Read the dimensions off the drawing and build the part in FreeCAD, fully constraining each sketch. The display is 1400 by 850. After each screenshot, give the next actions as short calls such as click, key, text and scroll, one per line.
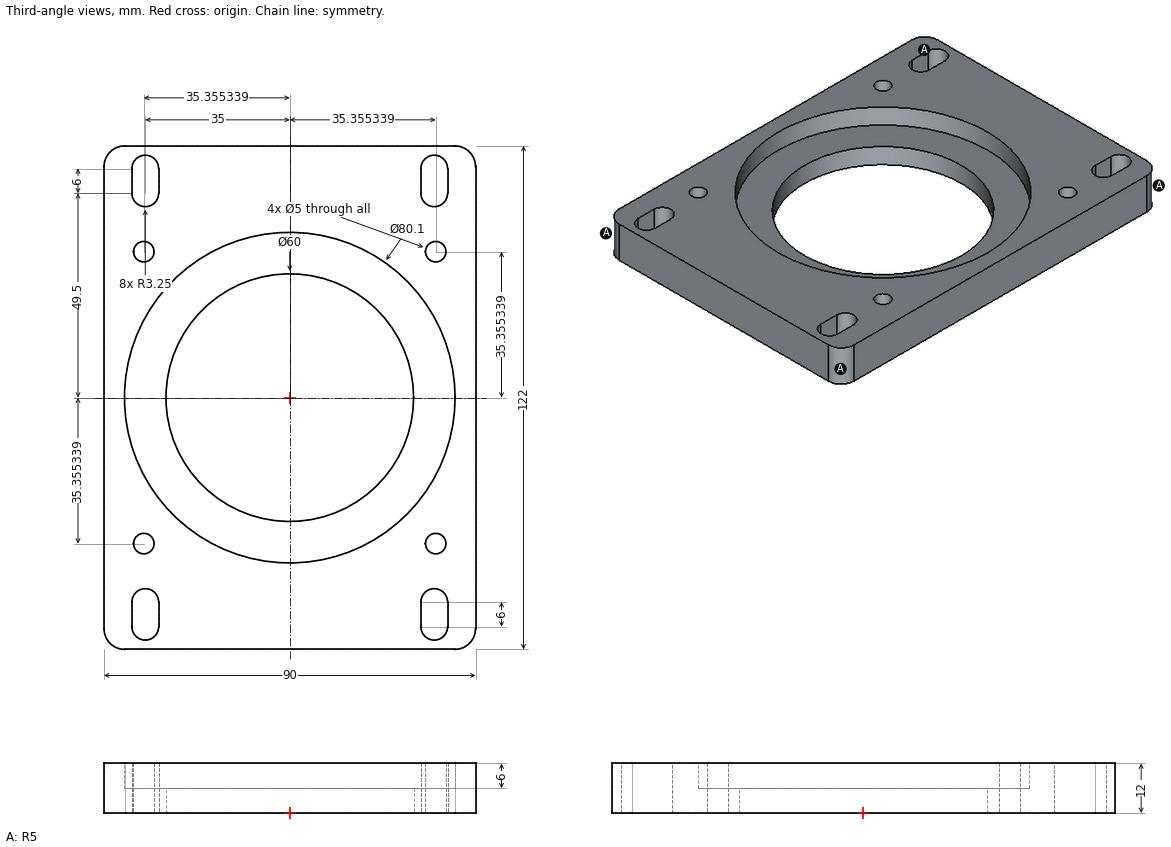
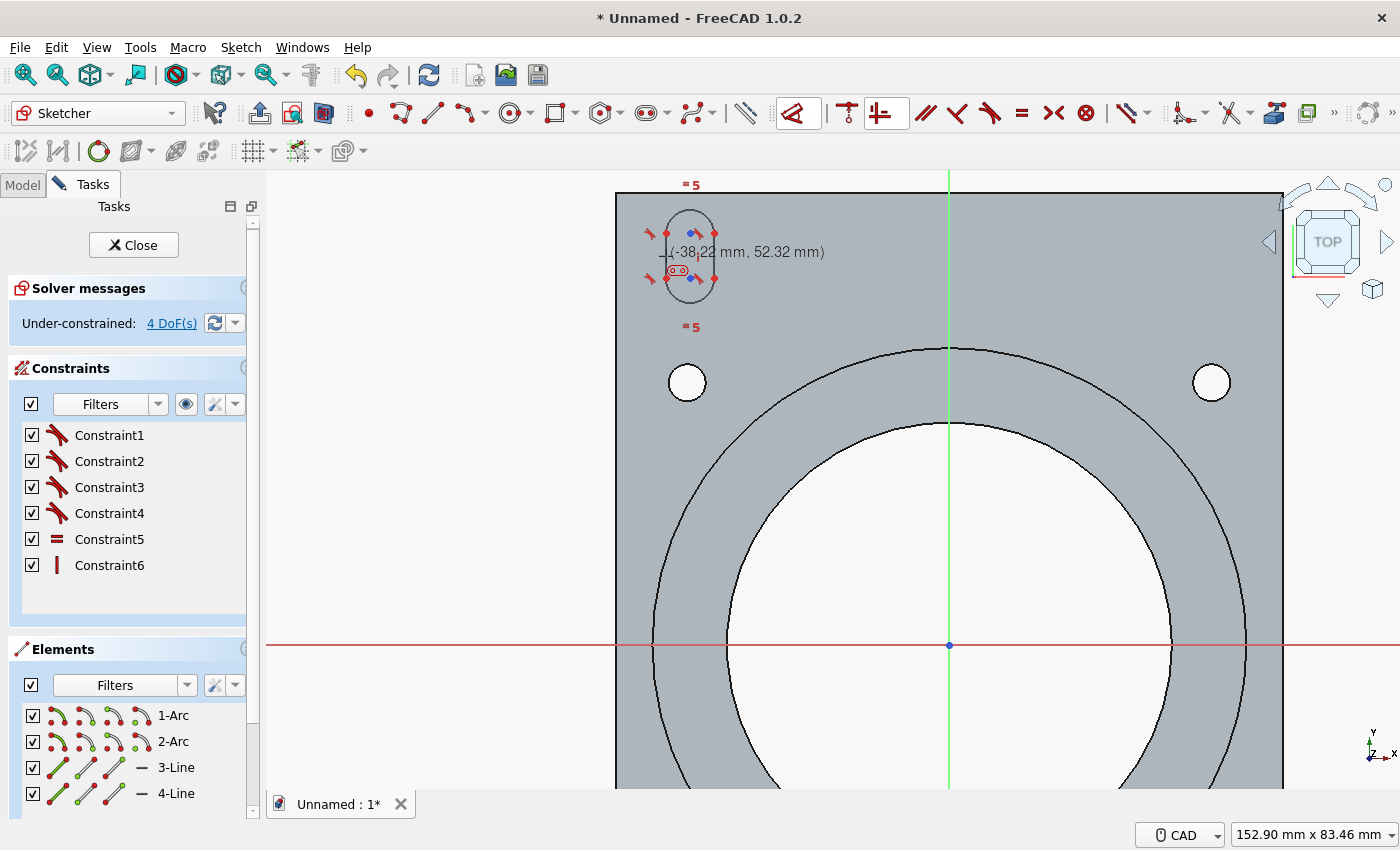
click(1209, 278)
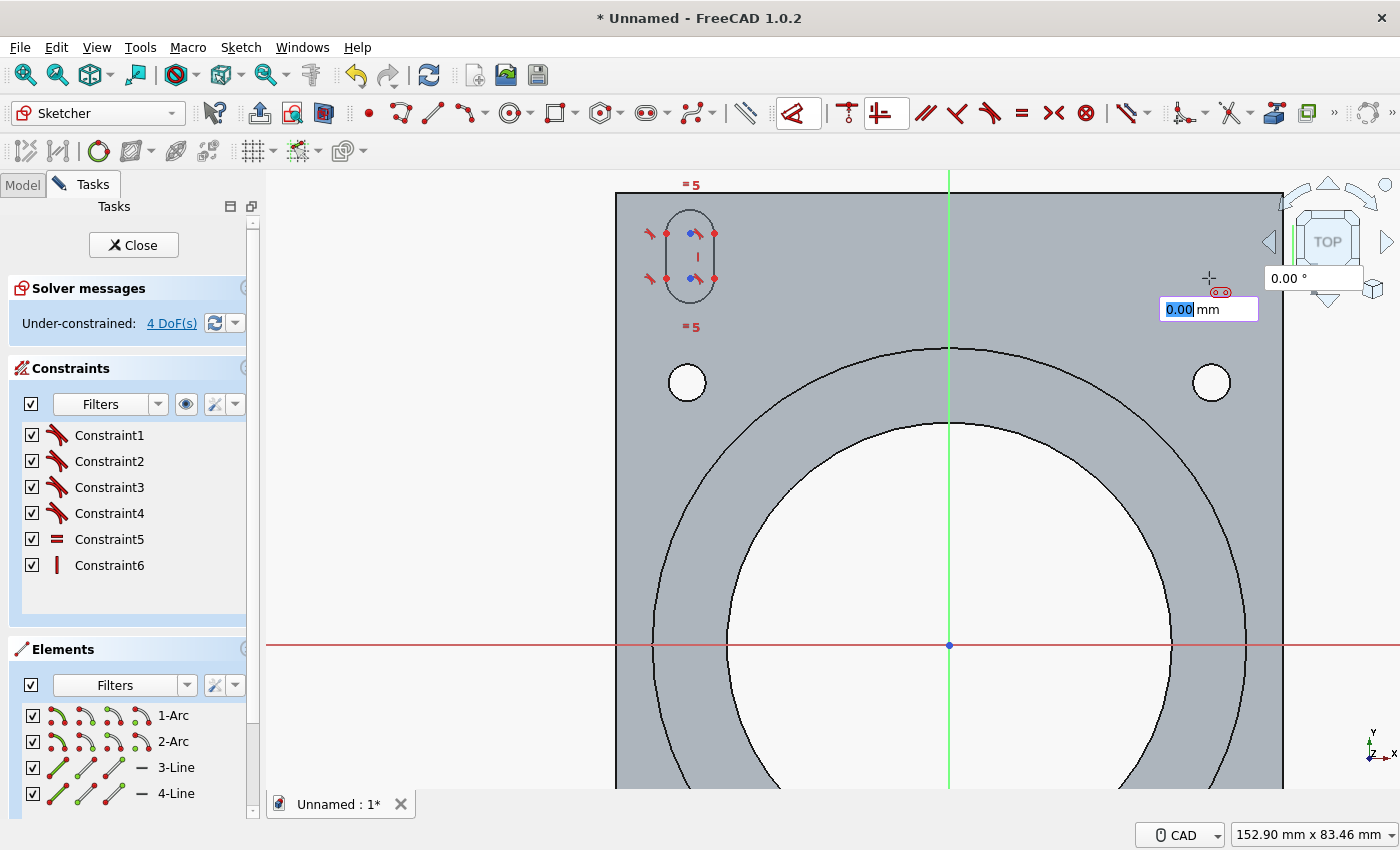
click(1209, 233)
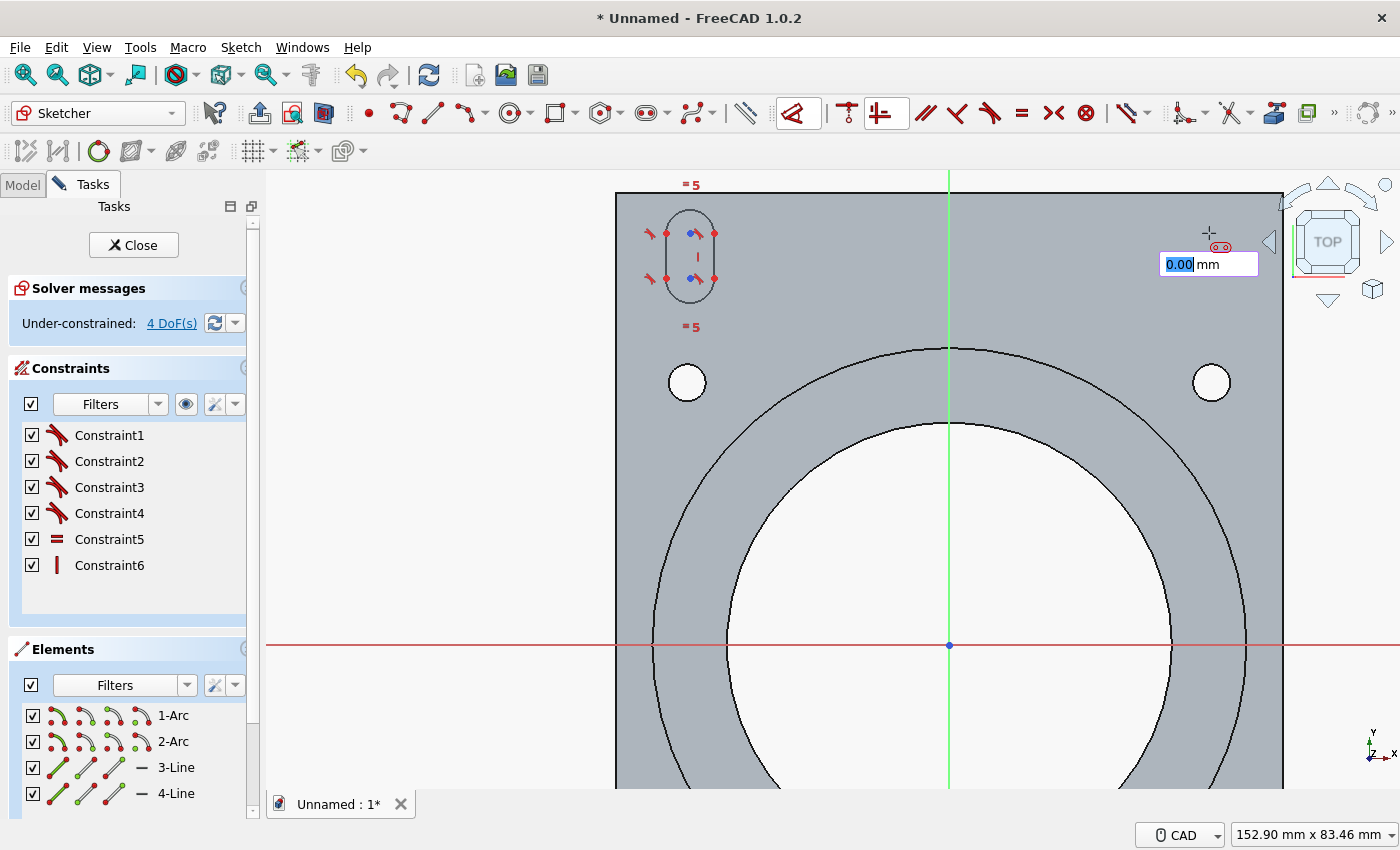
click(1233, 256)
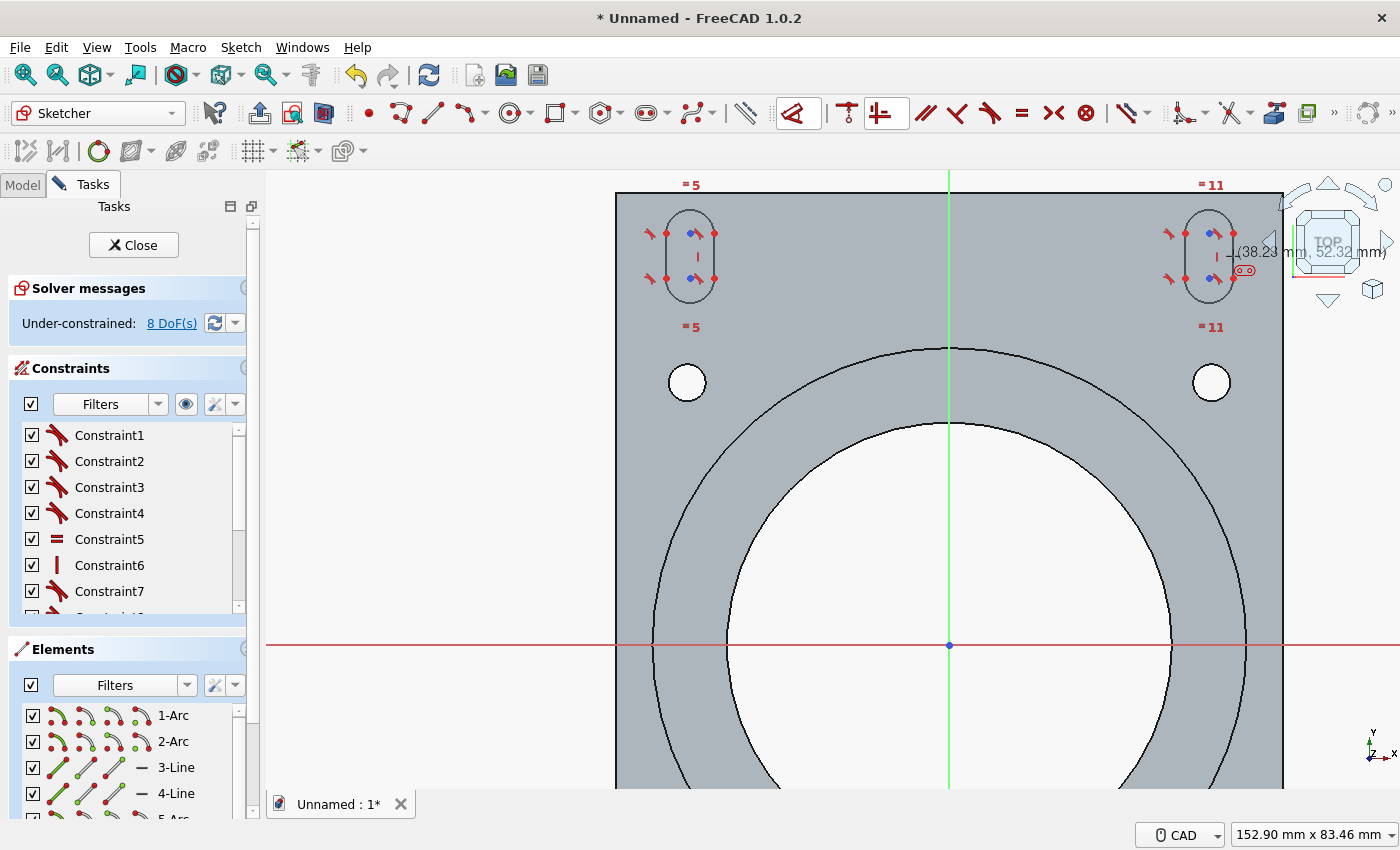
scroll(614, 344, down, 4)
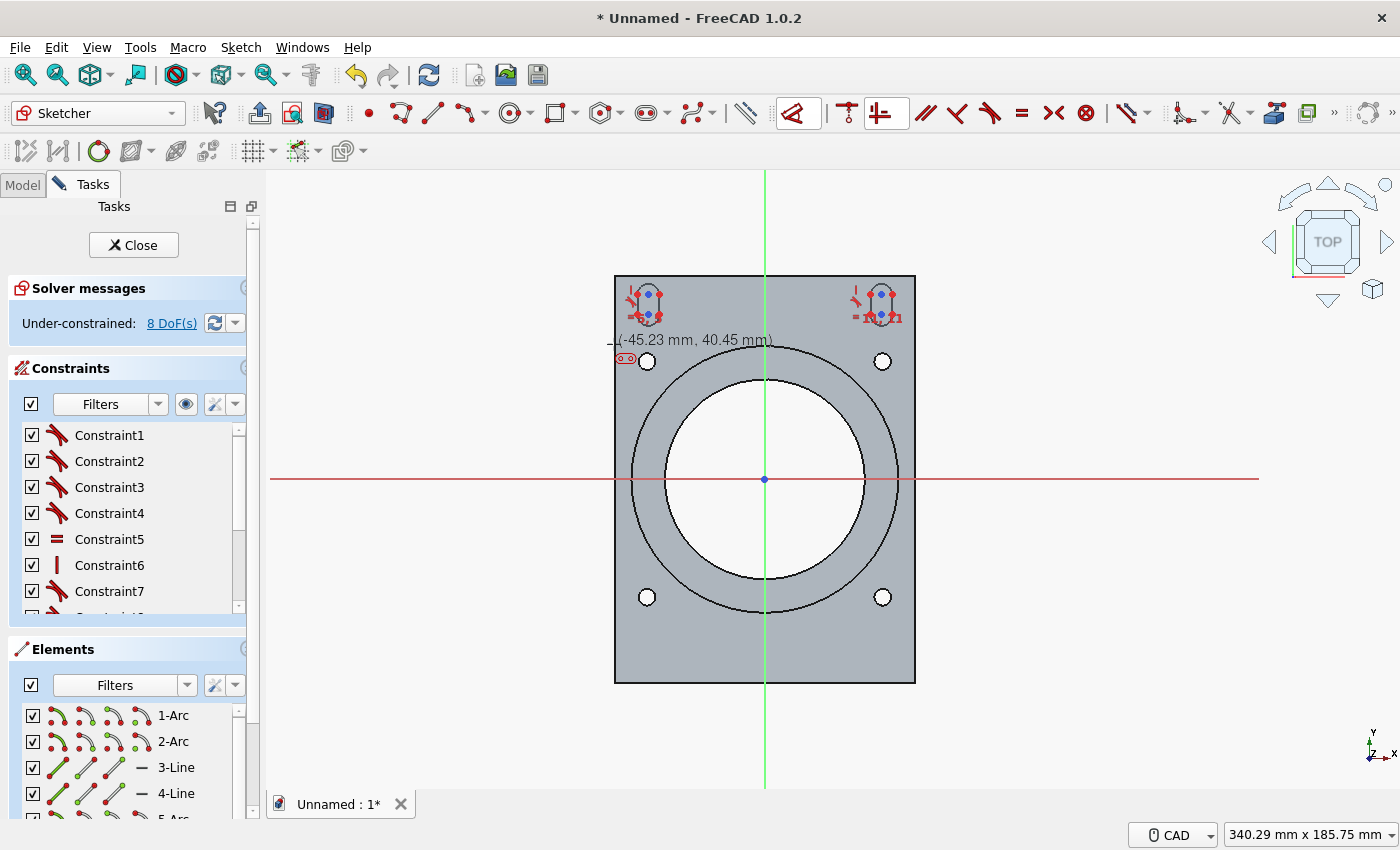
scroll(882, 664, up, 4)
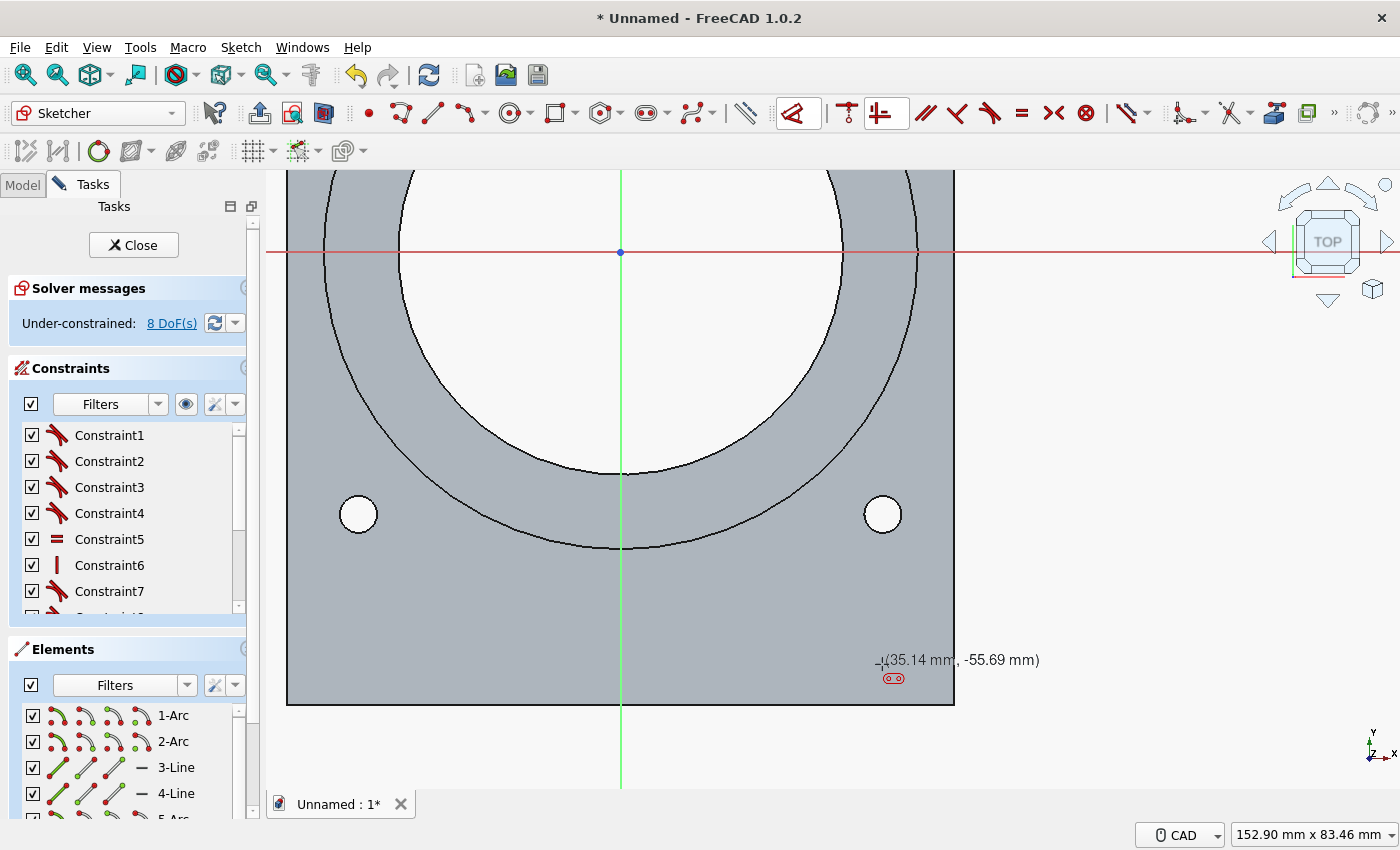
click(880, 664)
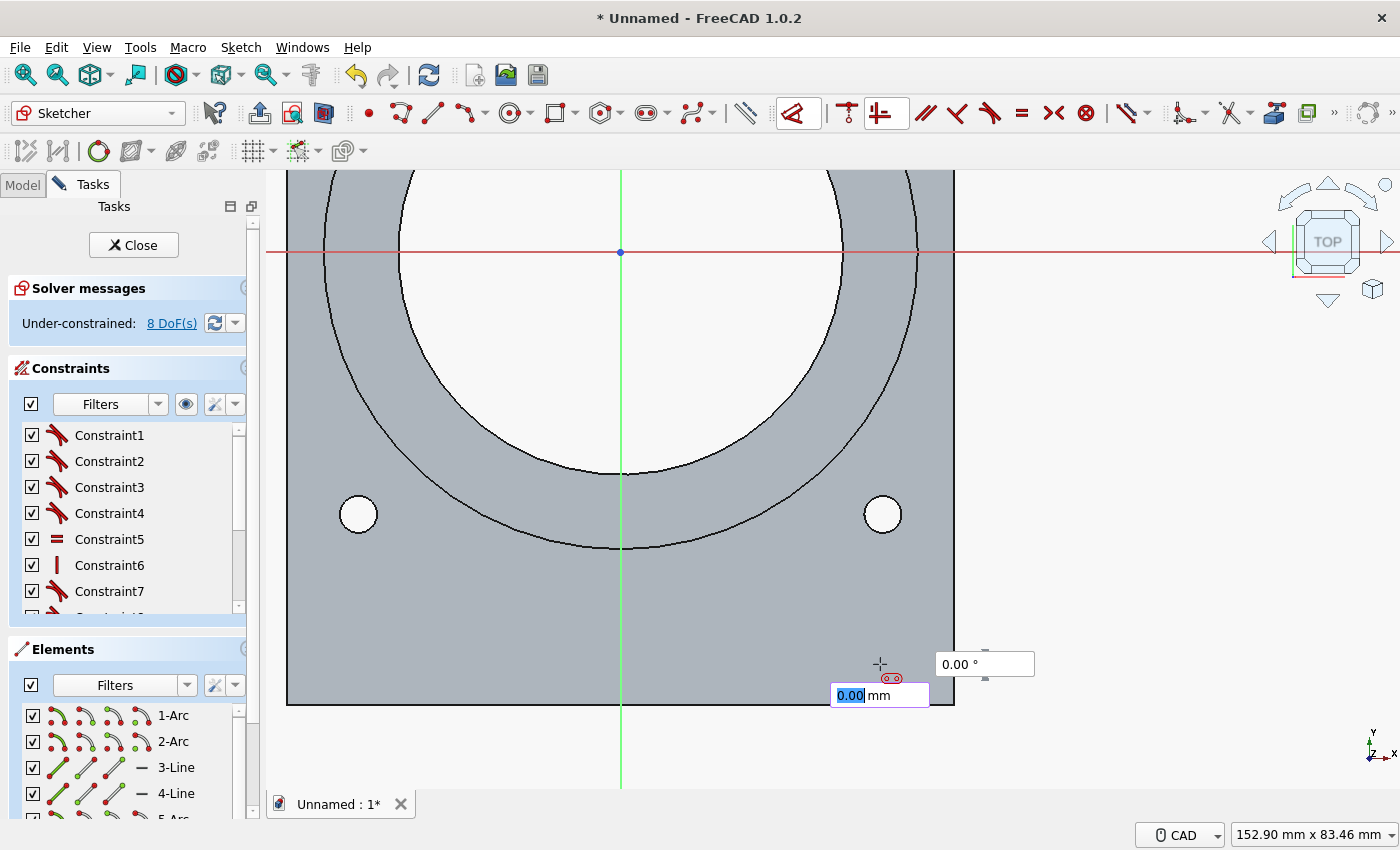
click(880, 619)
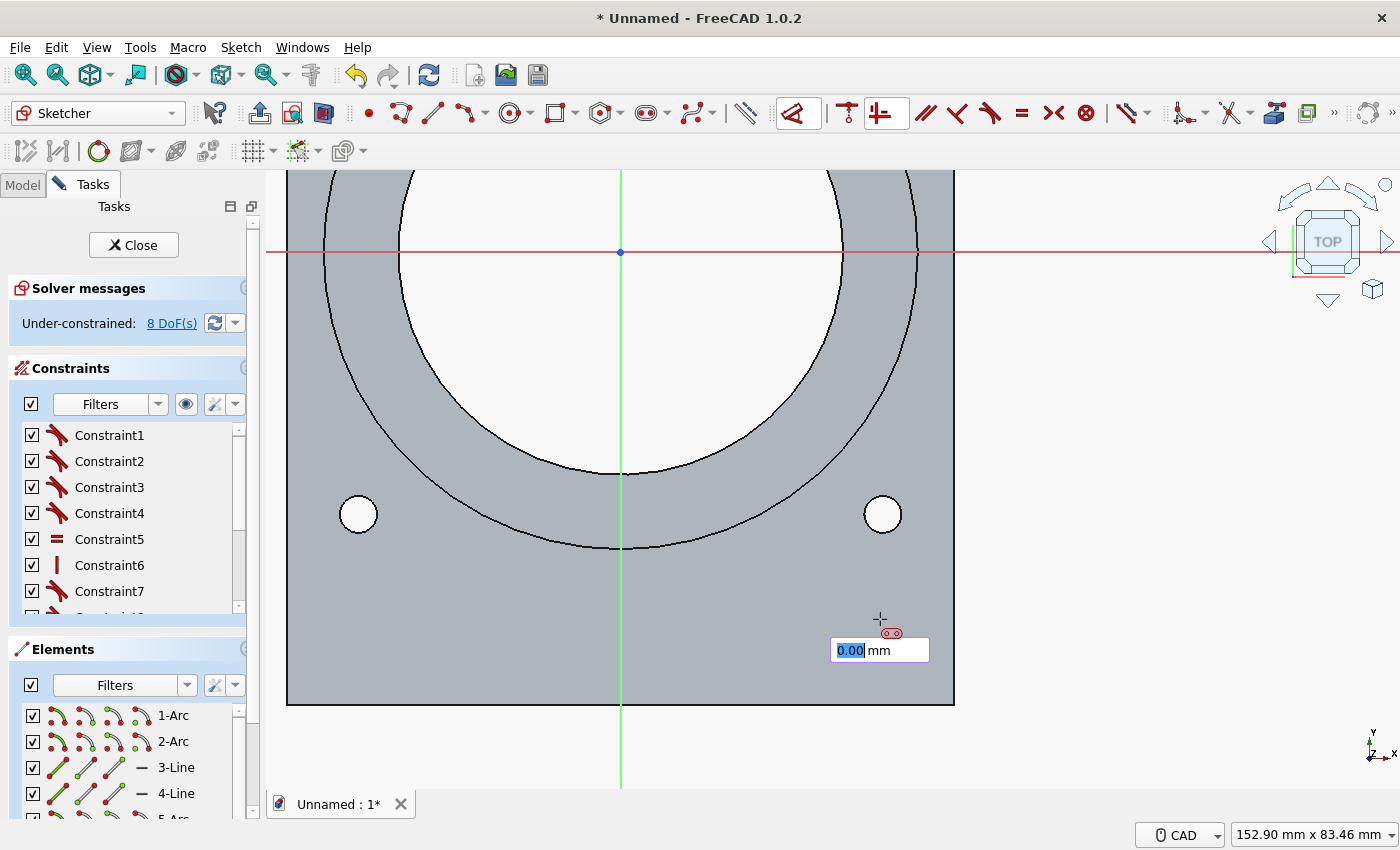
click(904, 642)